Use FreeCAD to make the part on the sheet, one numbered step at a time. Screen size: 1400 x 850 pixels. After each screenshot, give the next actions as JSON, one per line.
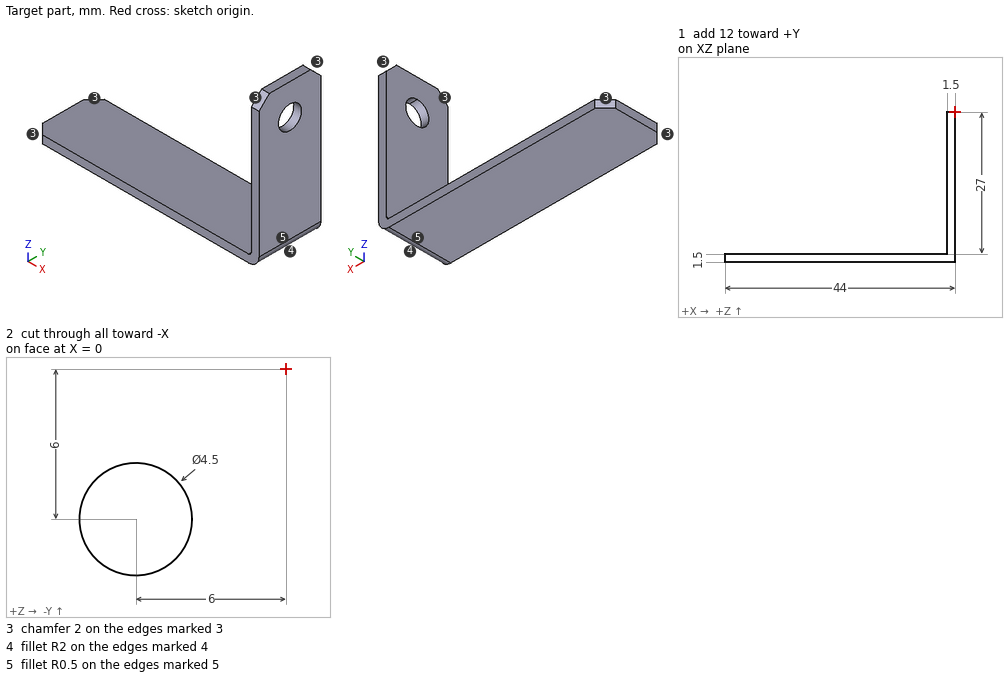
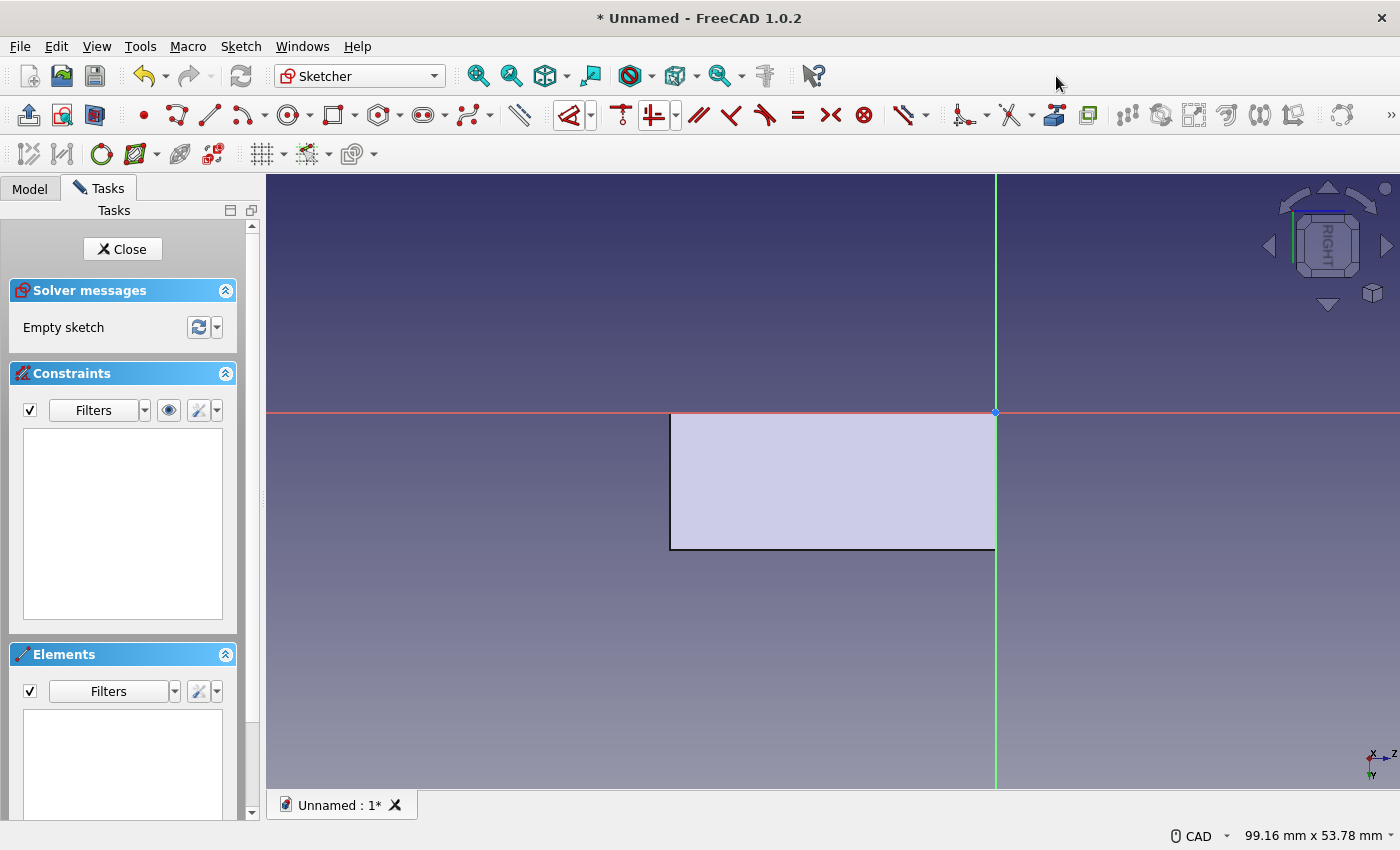
{"action": "scroll", "coordinate": [1009, 453], "scroll_direction": "up", "scroll_amount": 7}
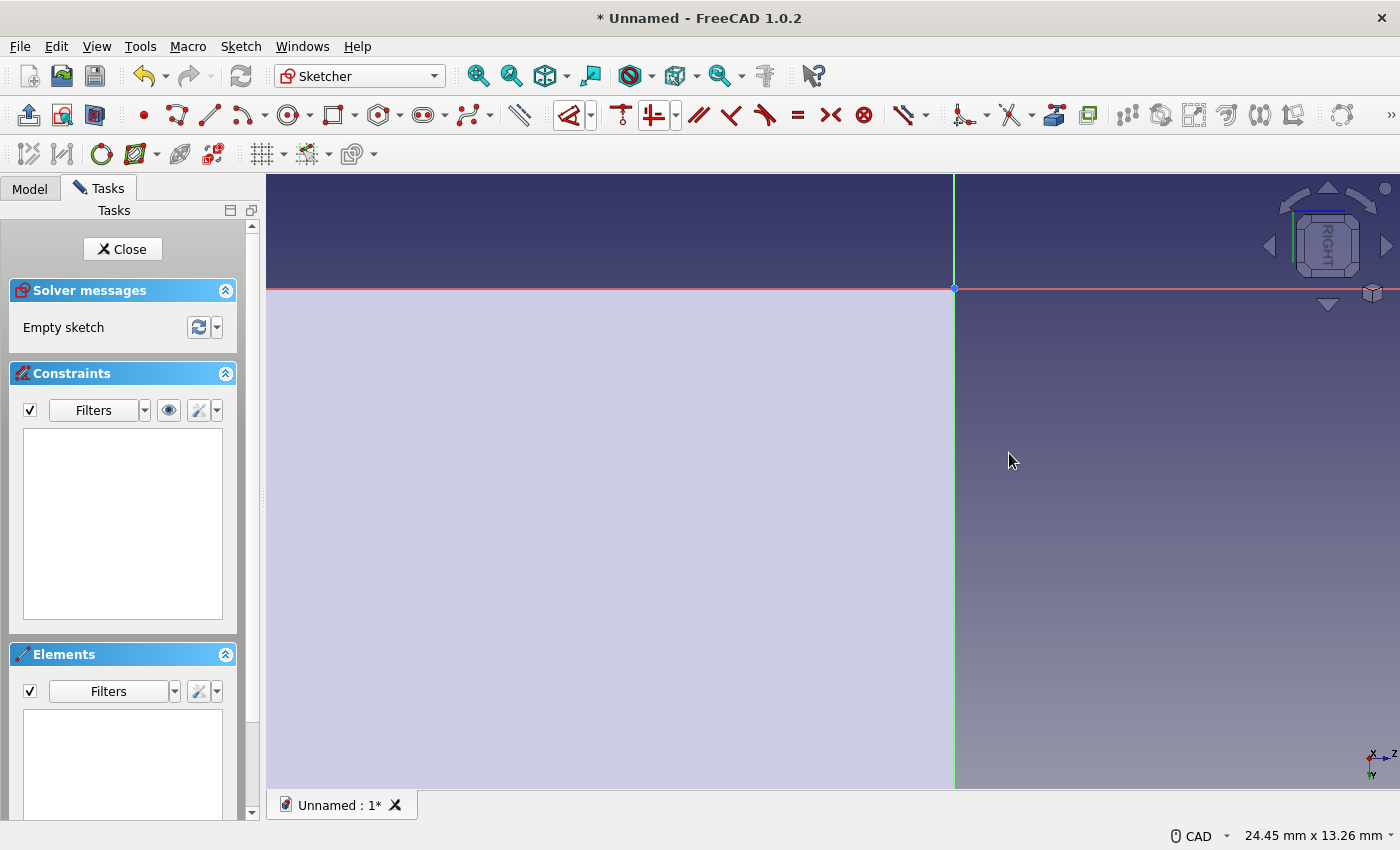
{"action": "key", "text": "g c"}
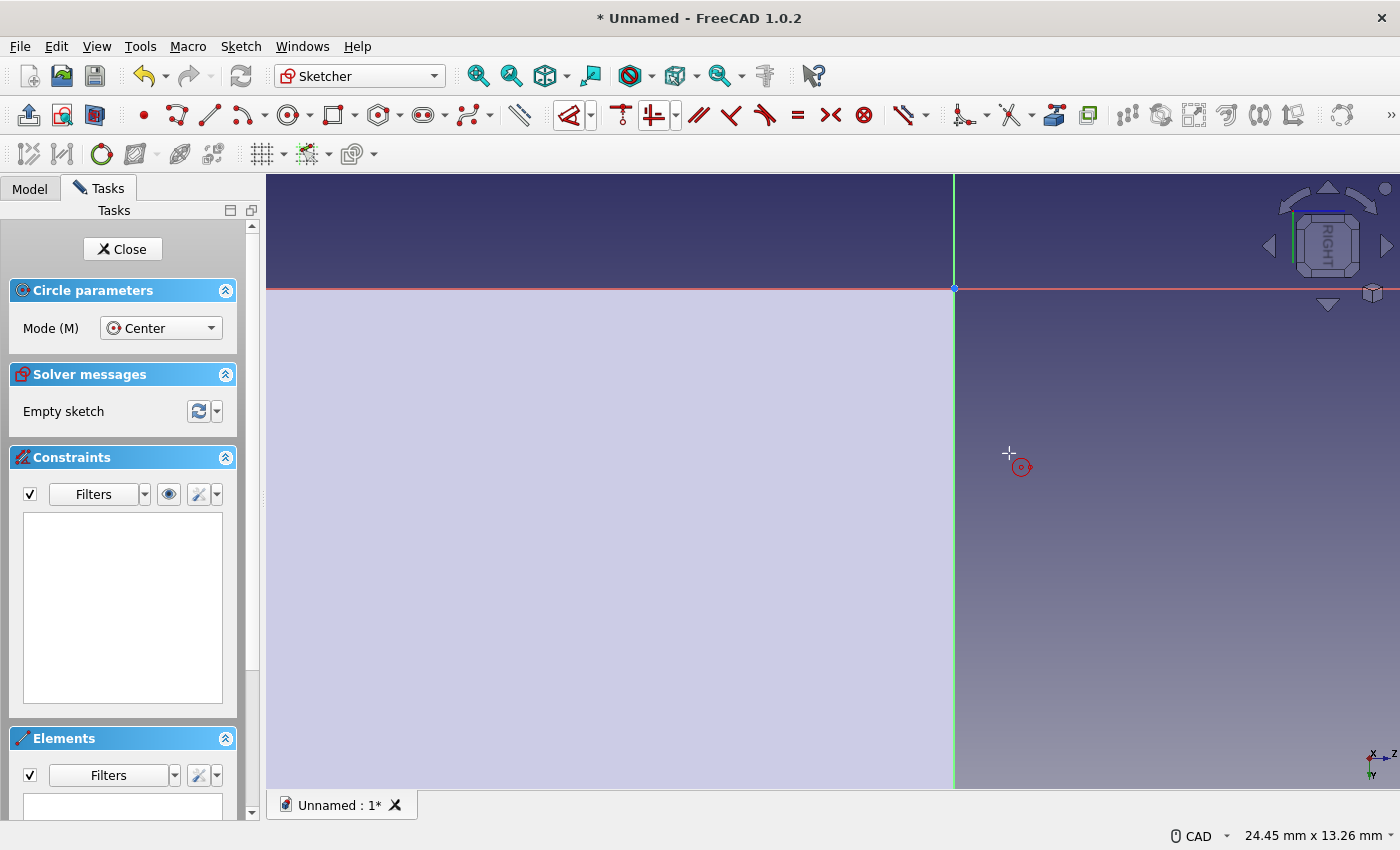
{"action": "left_click", "coordinate": [676, 567]}
{"action": "left_click", "coordinate": [750, 493]}
{"action": "key", "text": "Escape"}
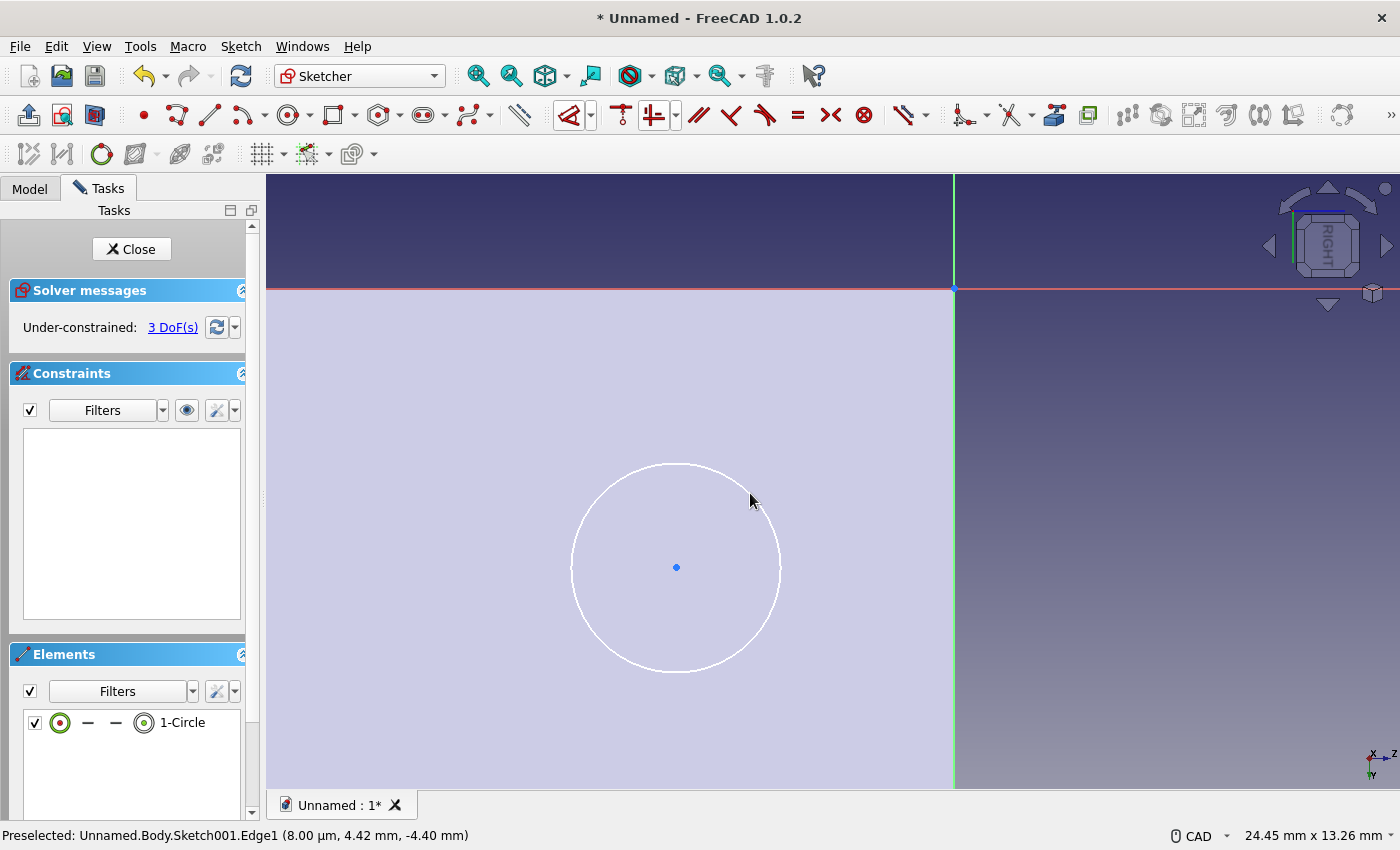
{"action": "left_click", "coordinate": [750, 494]}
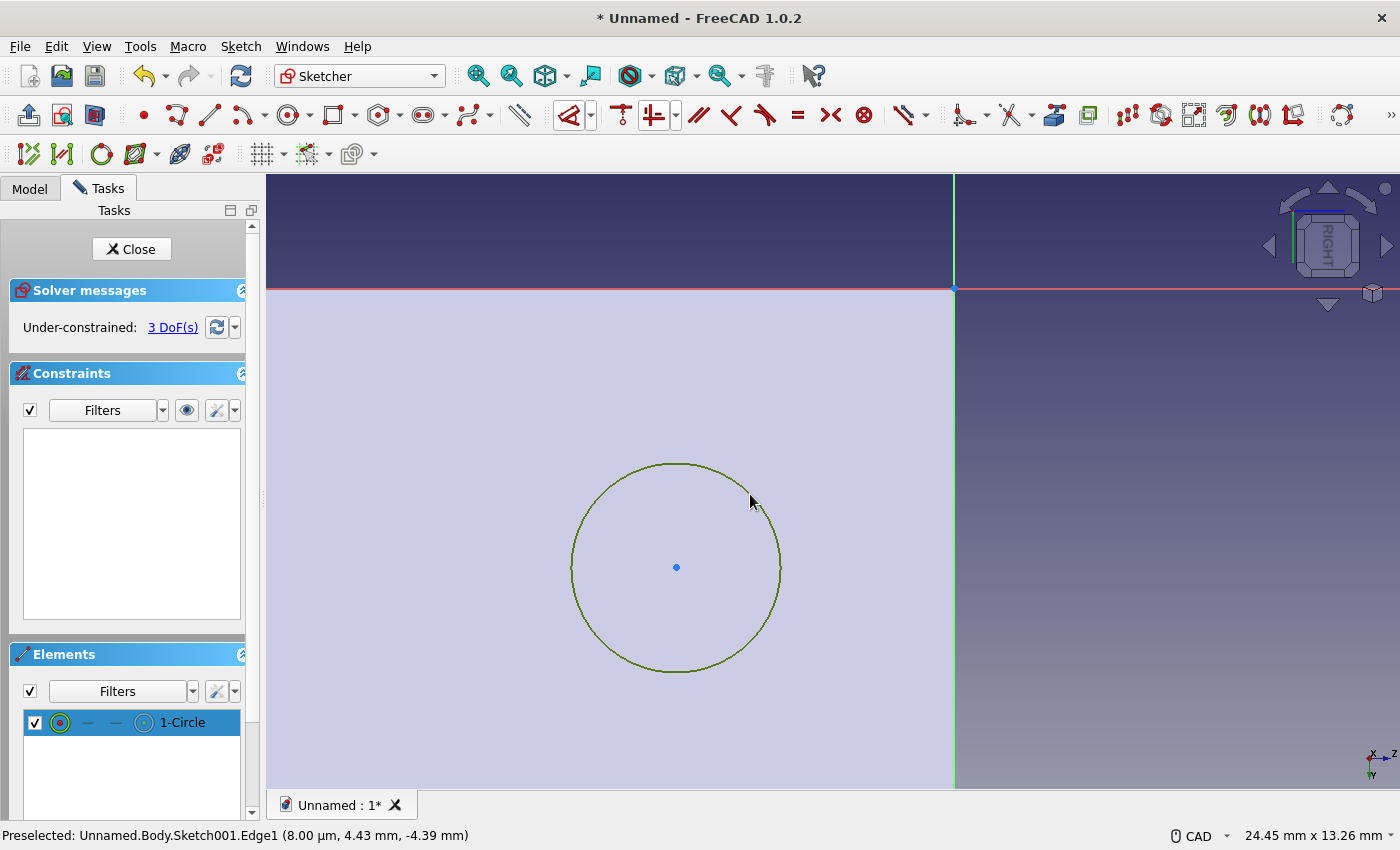
{"action": "key", "text": "k o"}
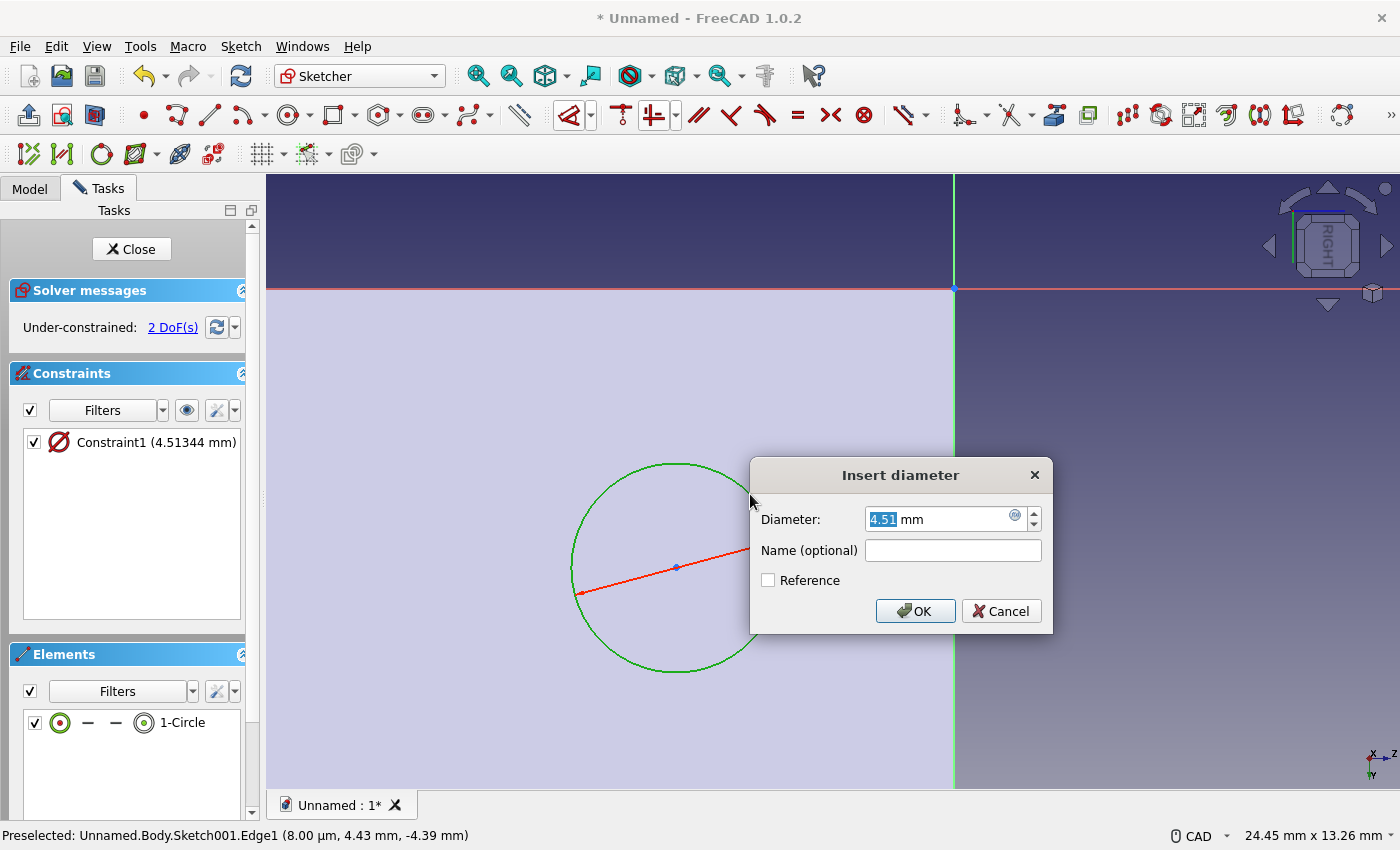
{"action": "type", "text": "4.5"}
{"action": "key", "text": "Return"}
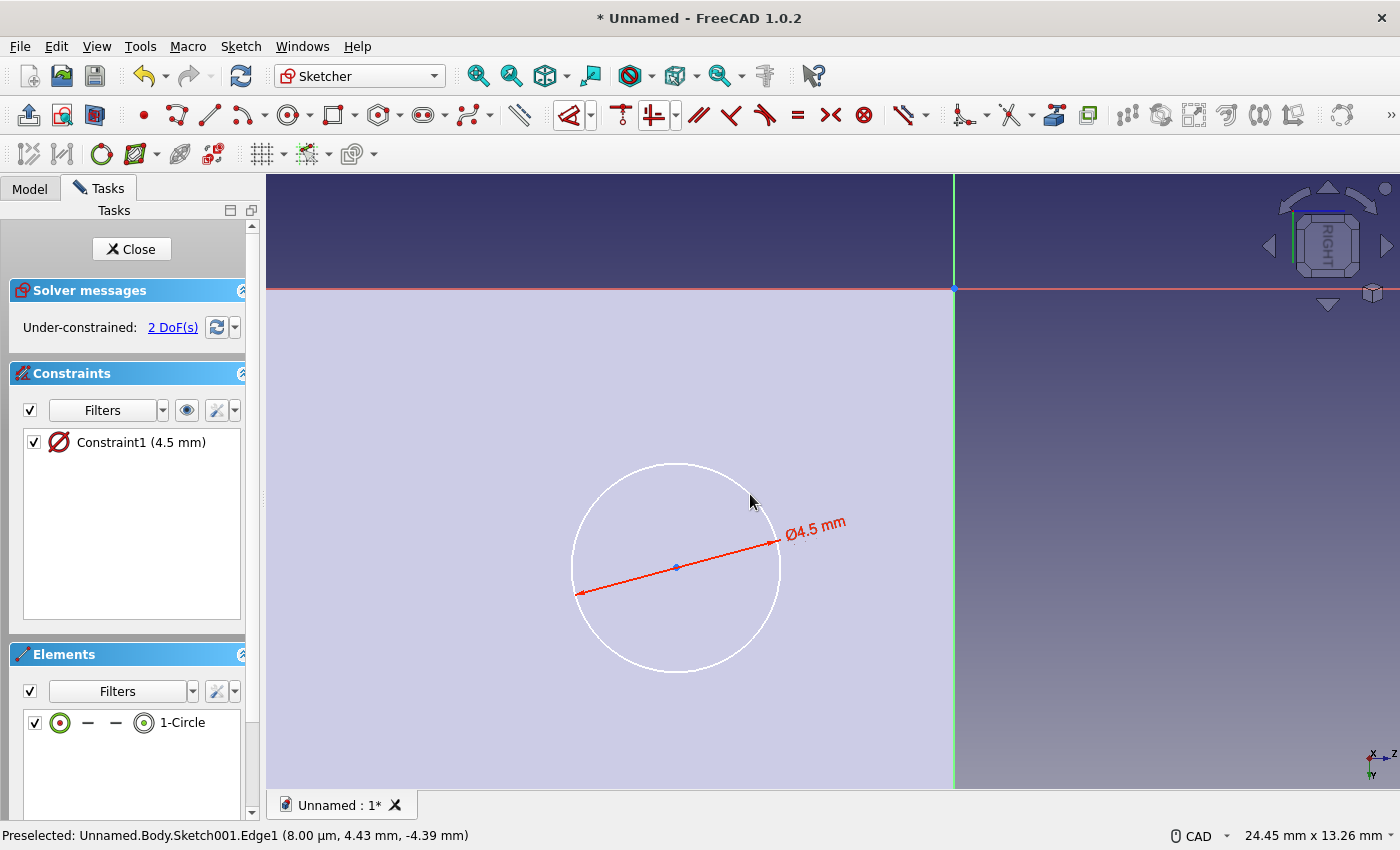
{"action": "left_click", "coordinate": [676, 568]}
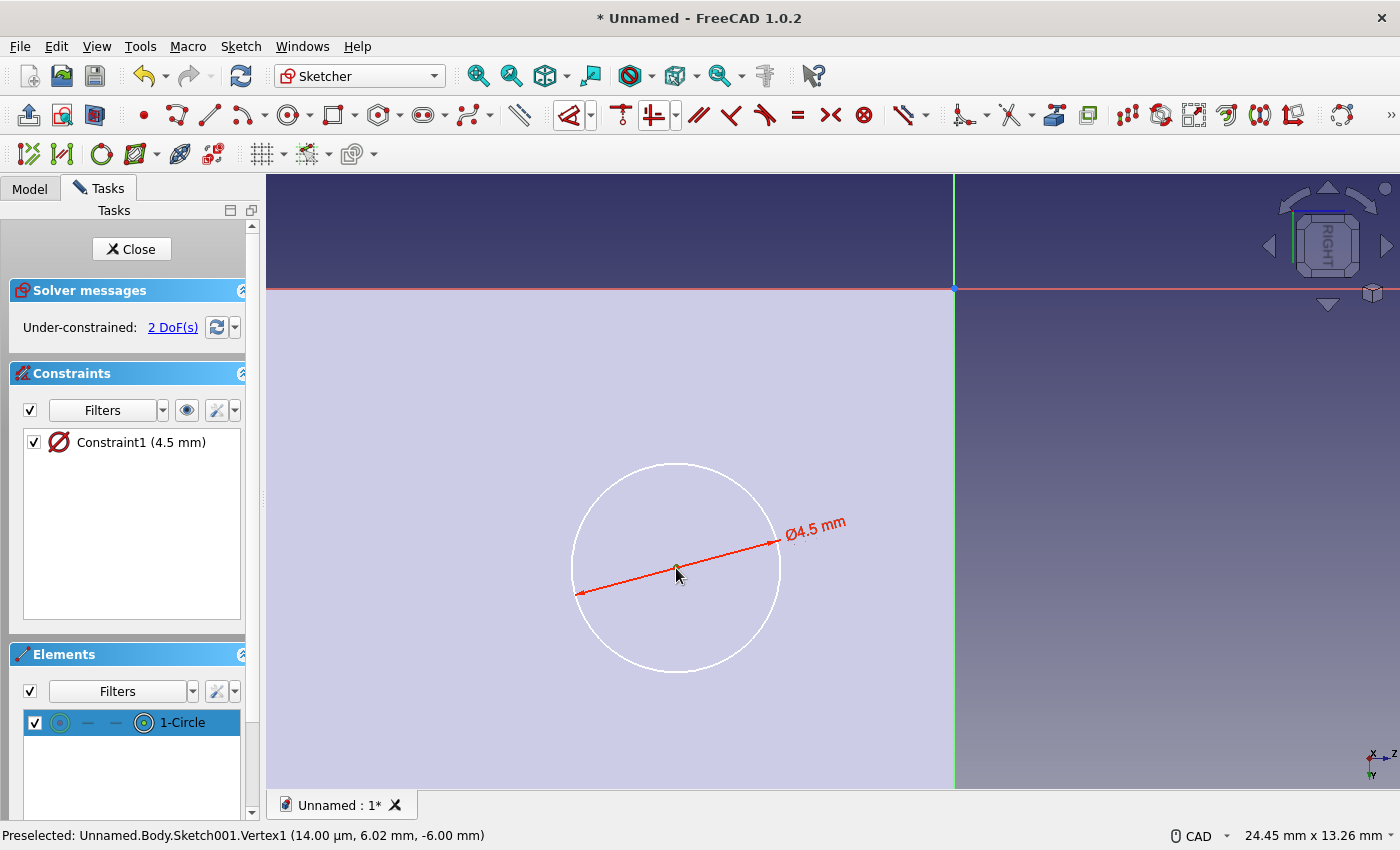
{"action": "key", "text": "l"}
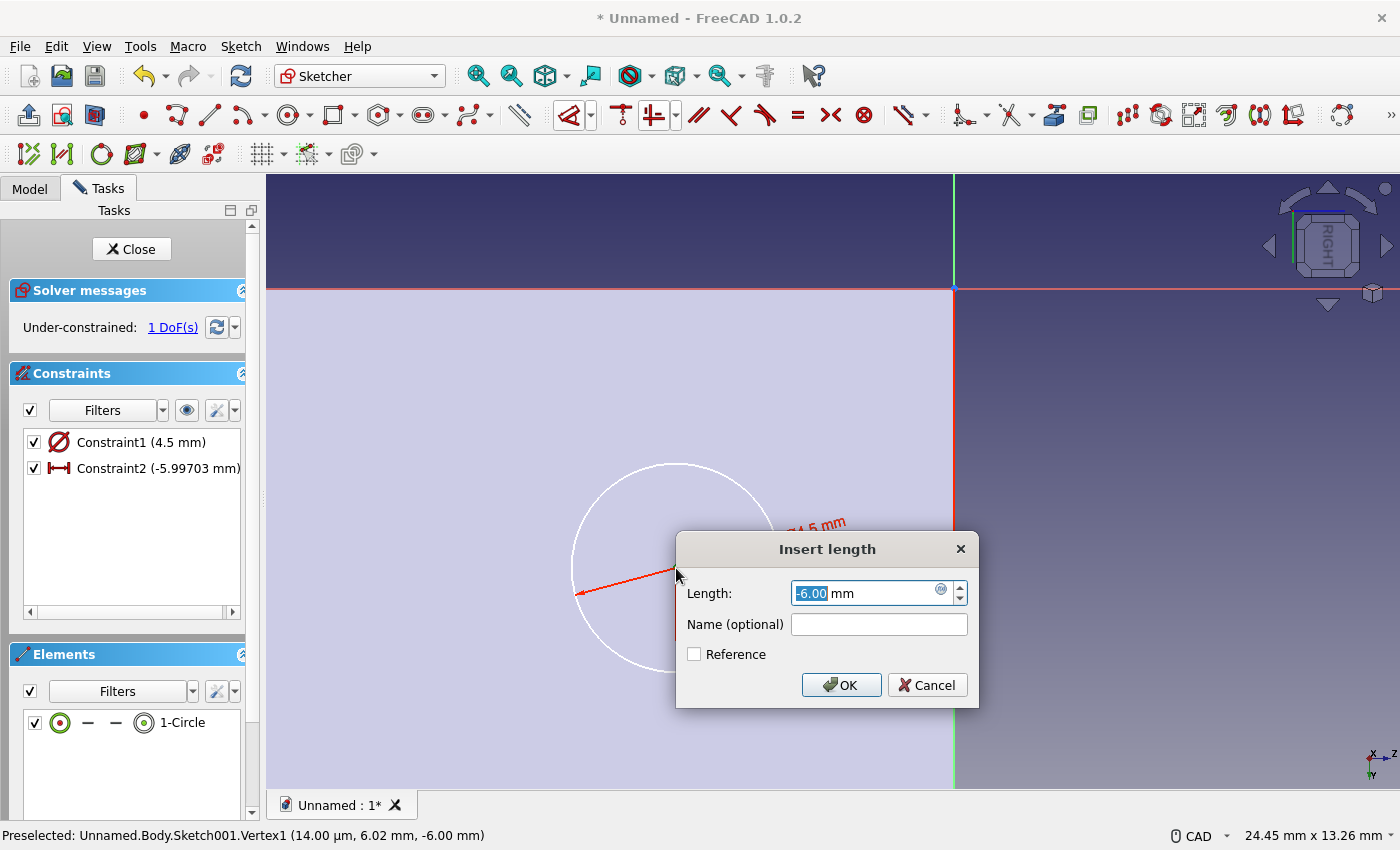
{"action": "type", "text": "-6"}
{"action": "key", "text": "Return"}